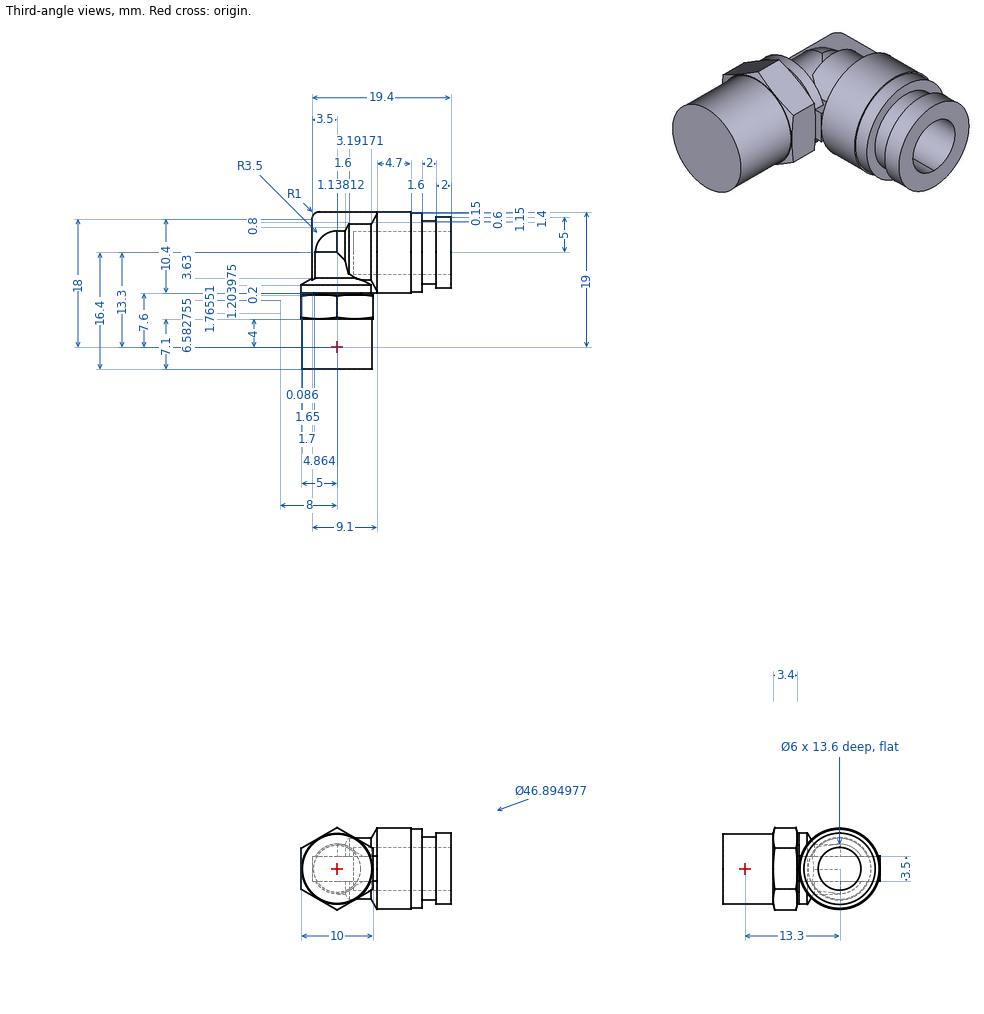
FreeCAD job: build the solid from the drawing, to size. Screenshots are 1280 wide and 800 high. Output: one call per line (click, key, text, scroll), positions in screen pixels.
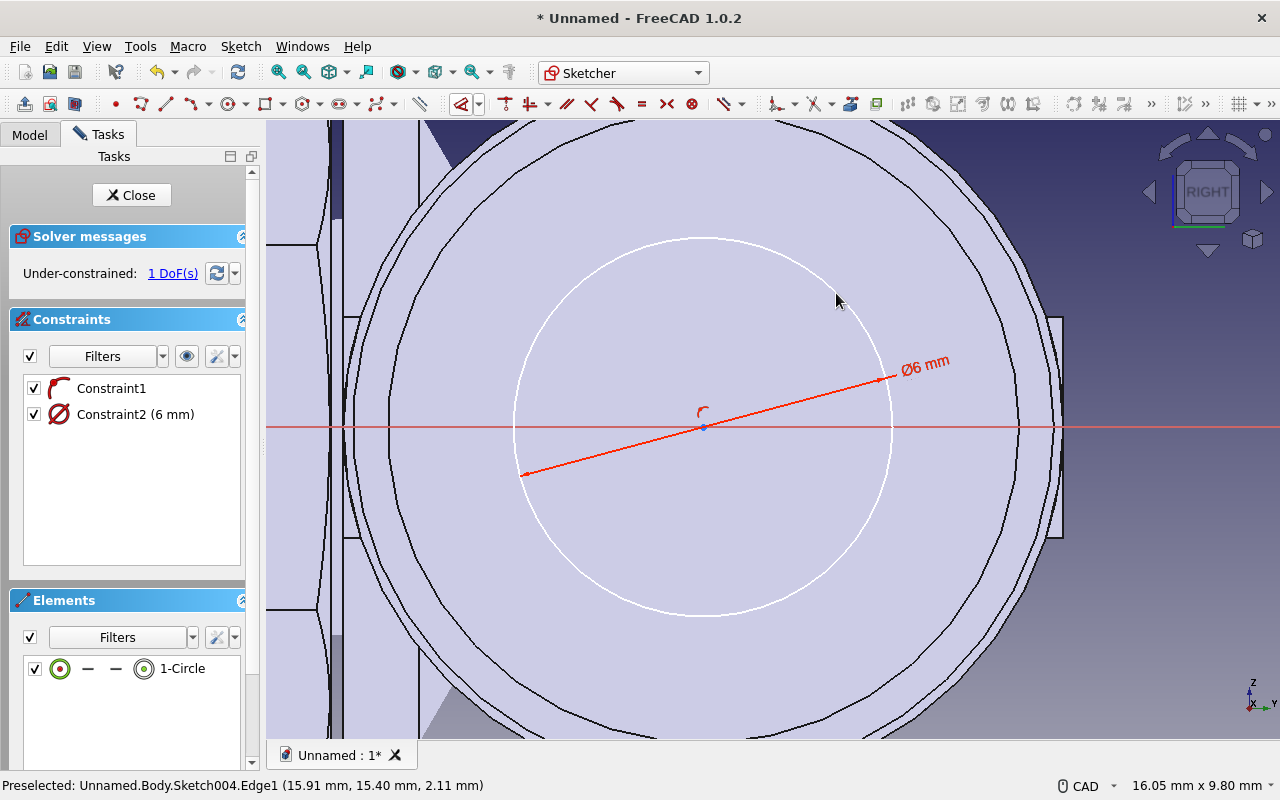
click(703, 427)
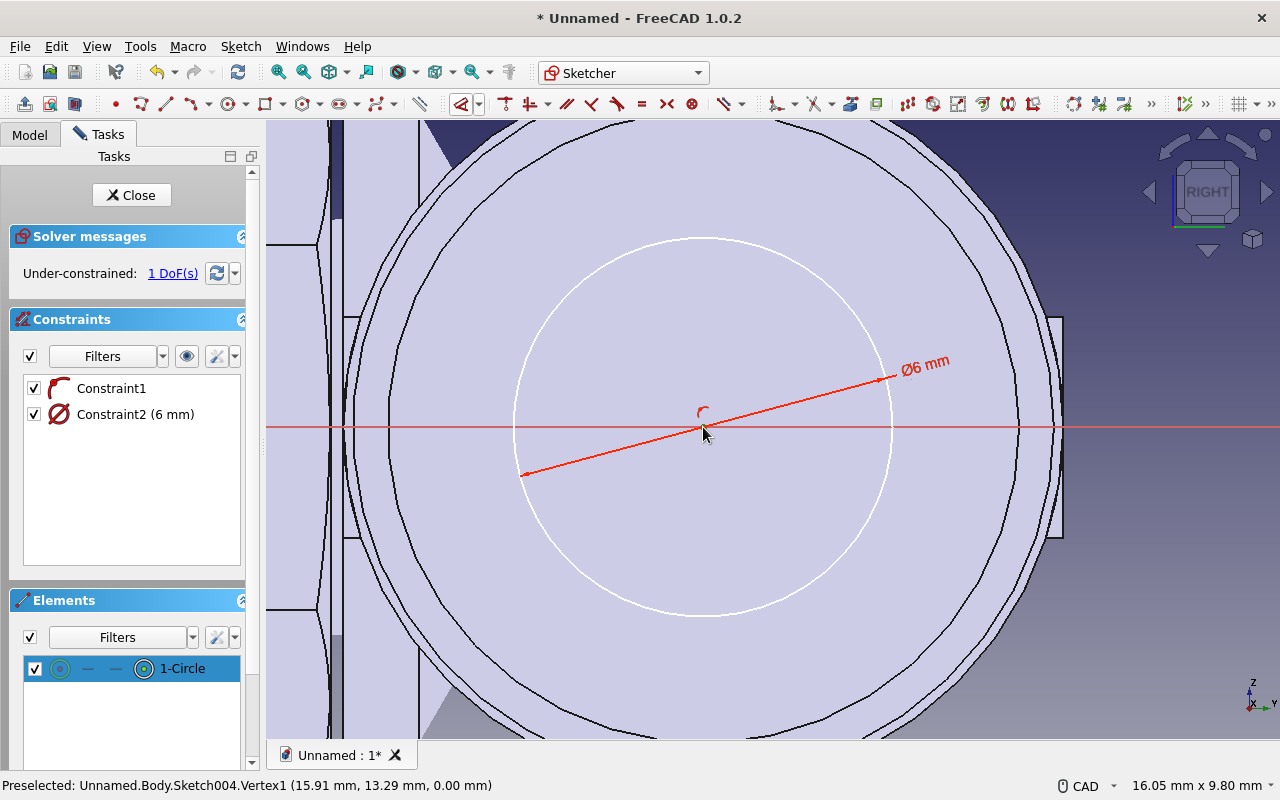
key(l)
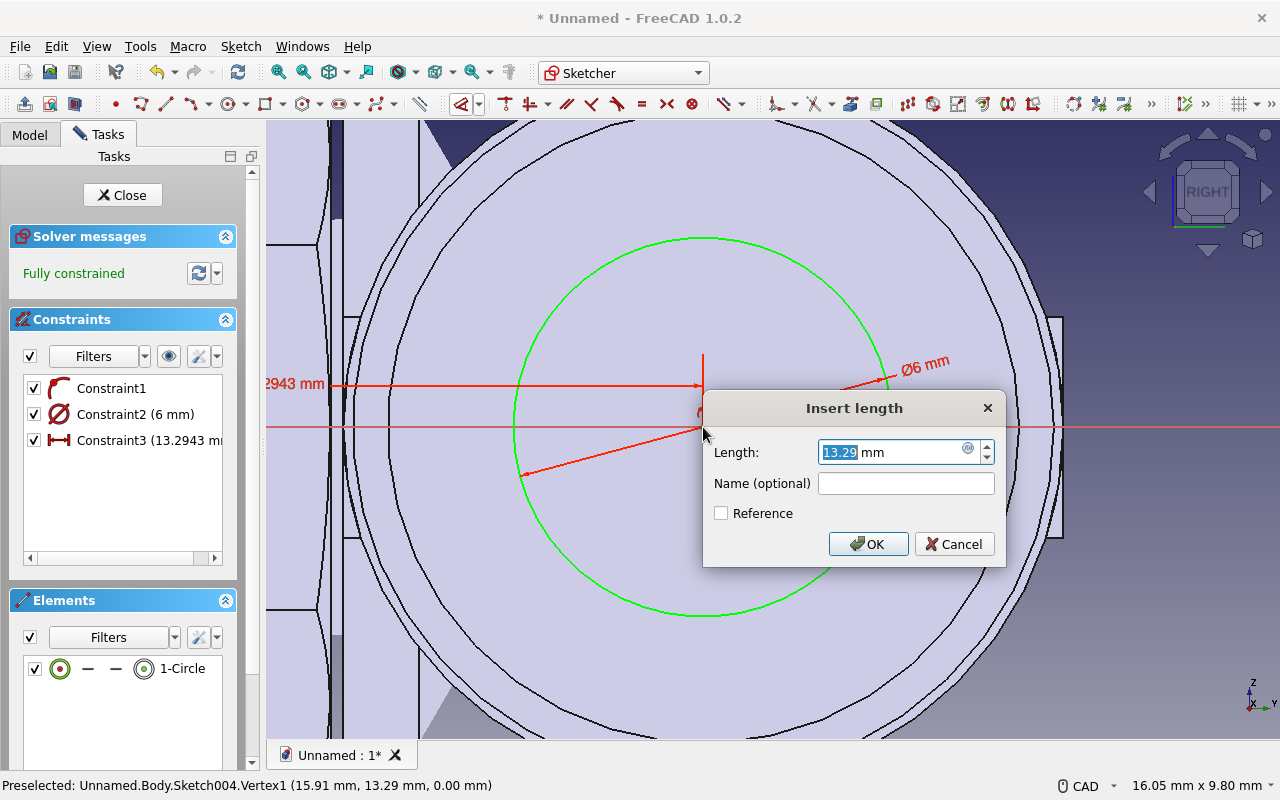
text(13.3)
key(Return)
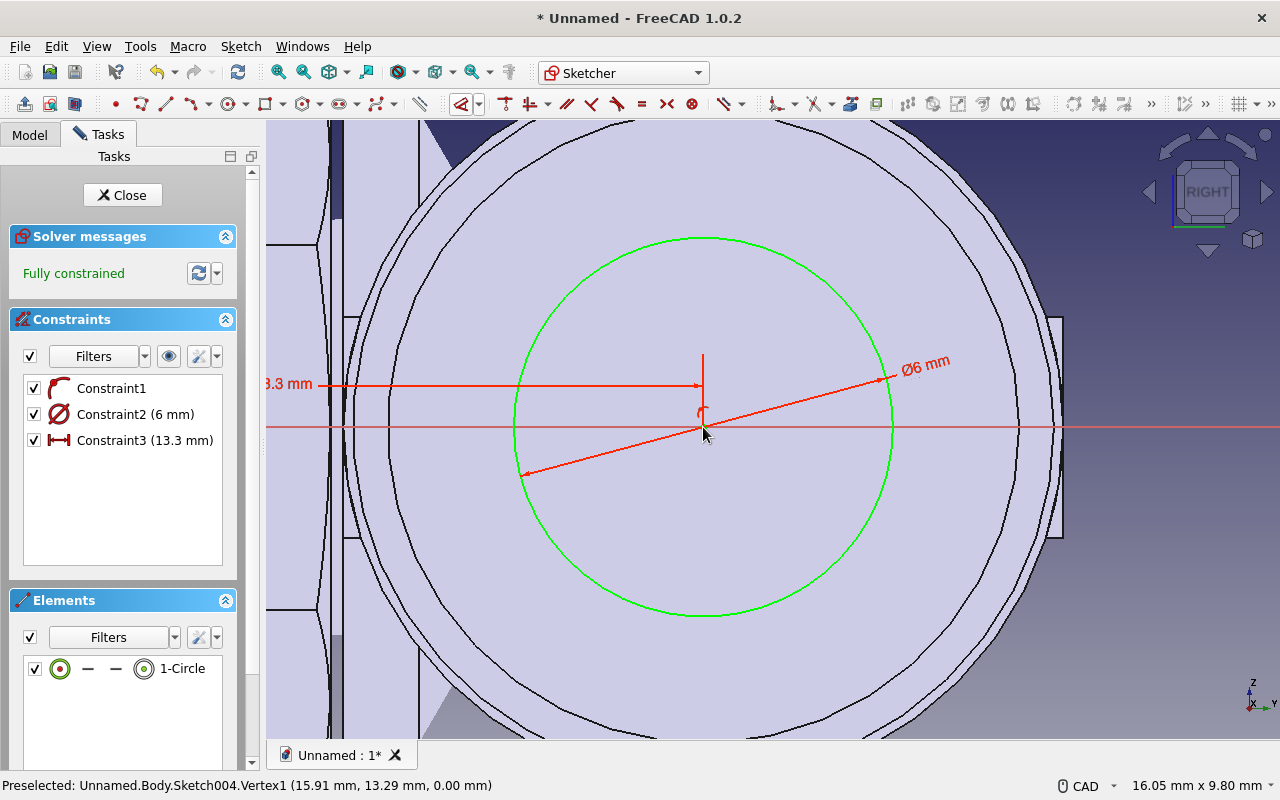
click(123, 195)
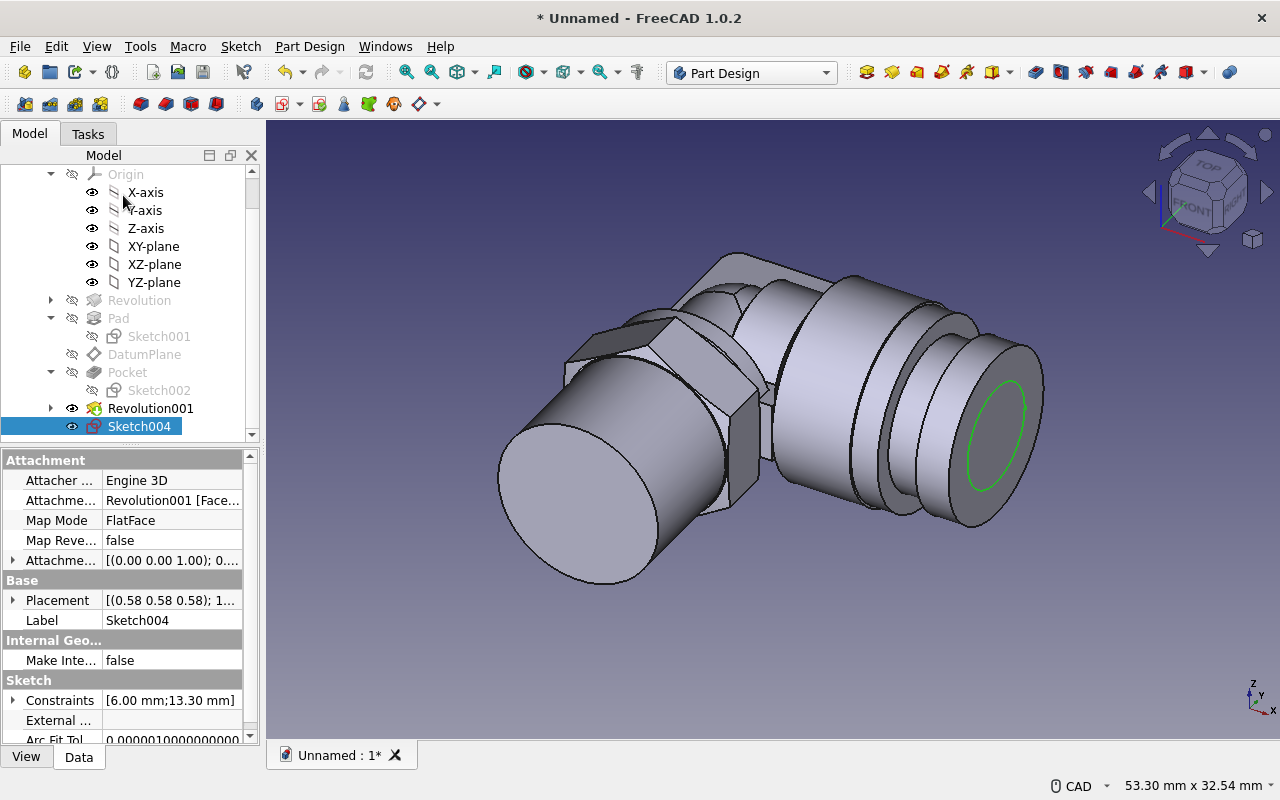
click(1061, 72)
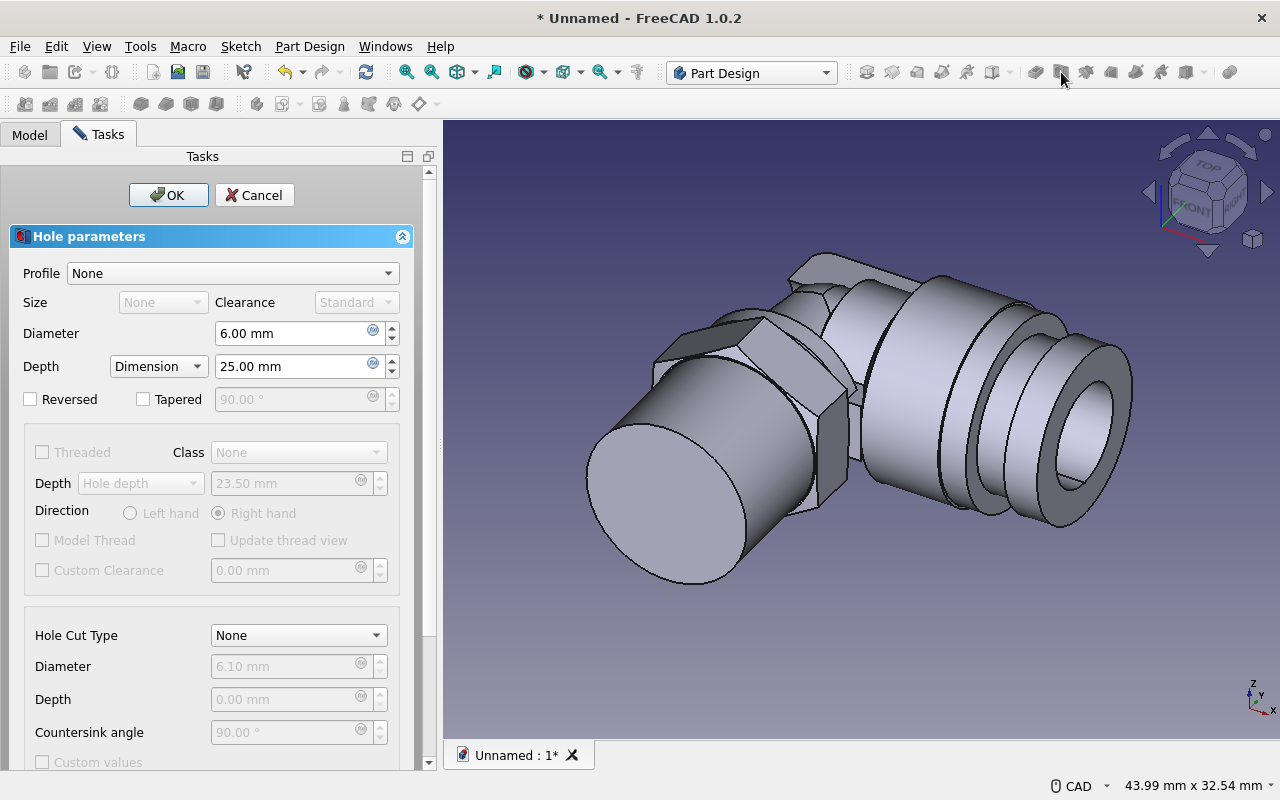
triple_click(300, 334)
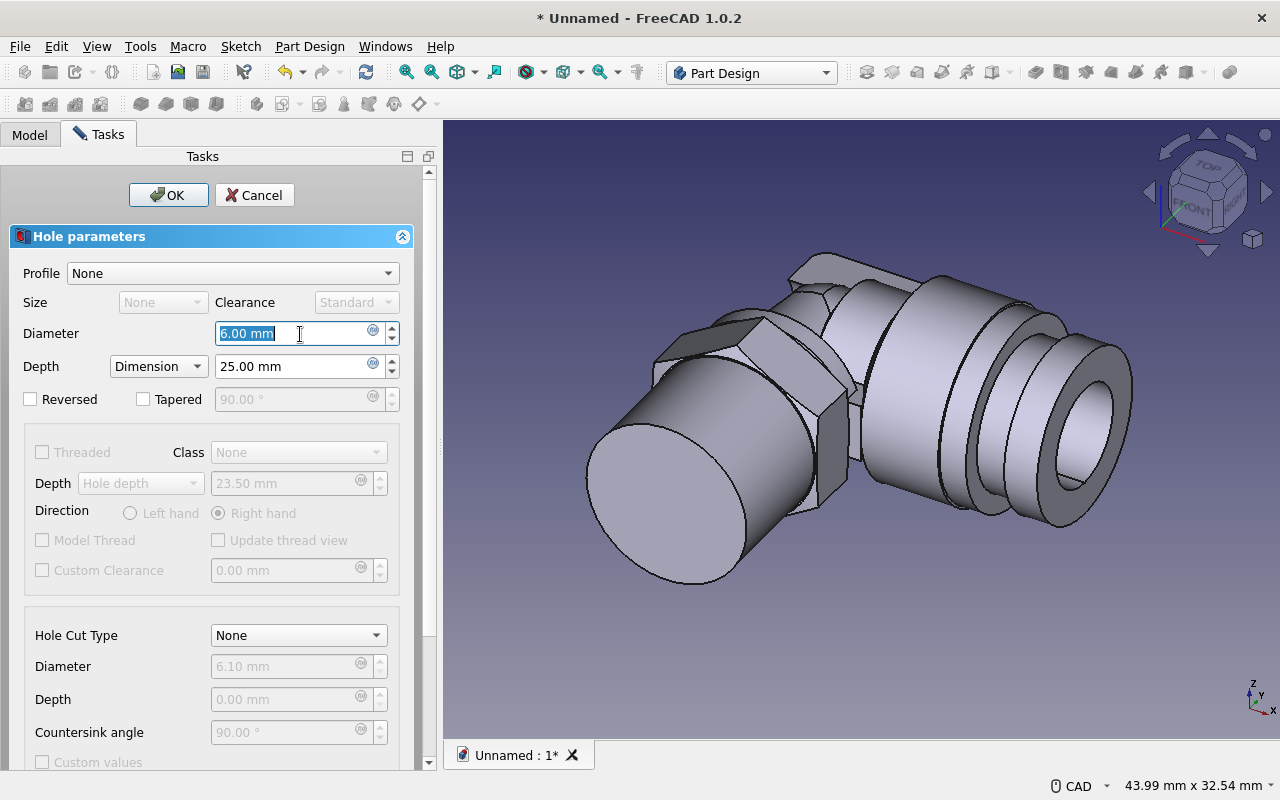
text(6)
key(Tab)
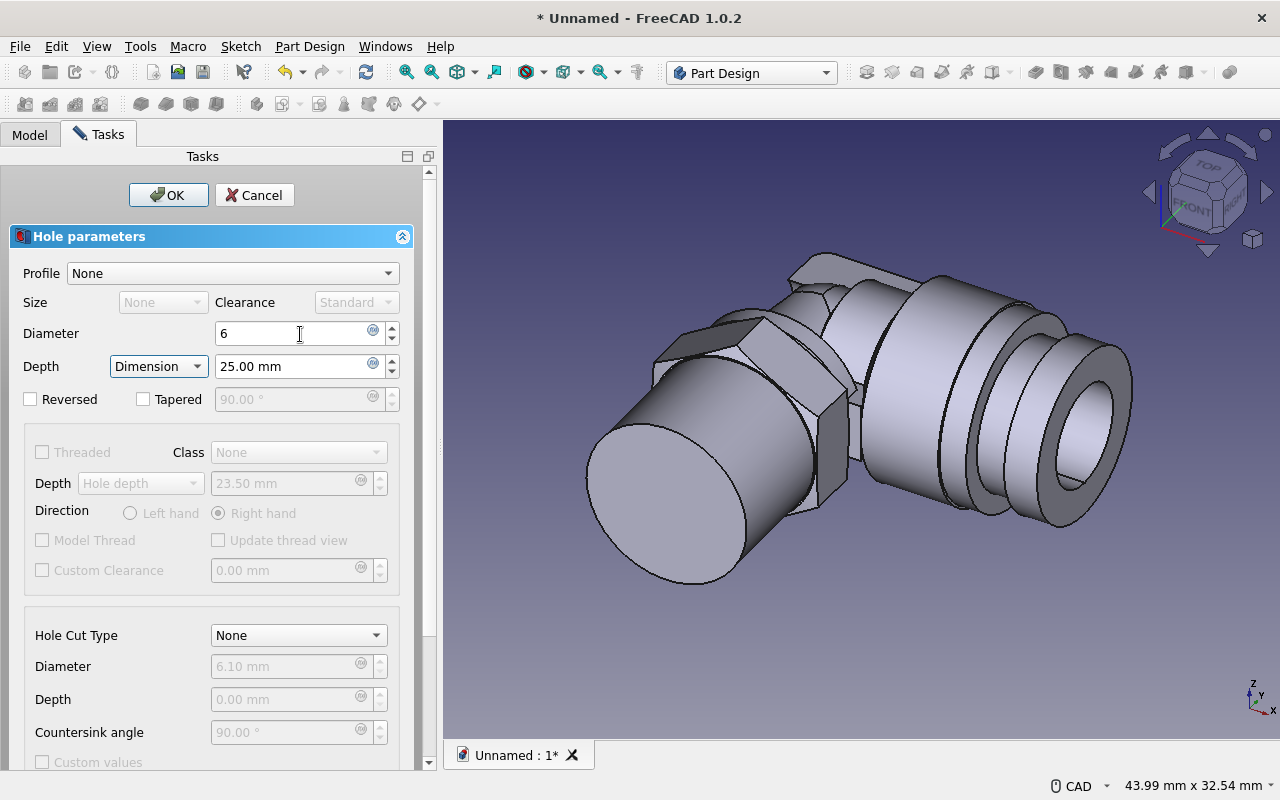
triple_click(300, 366)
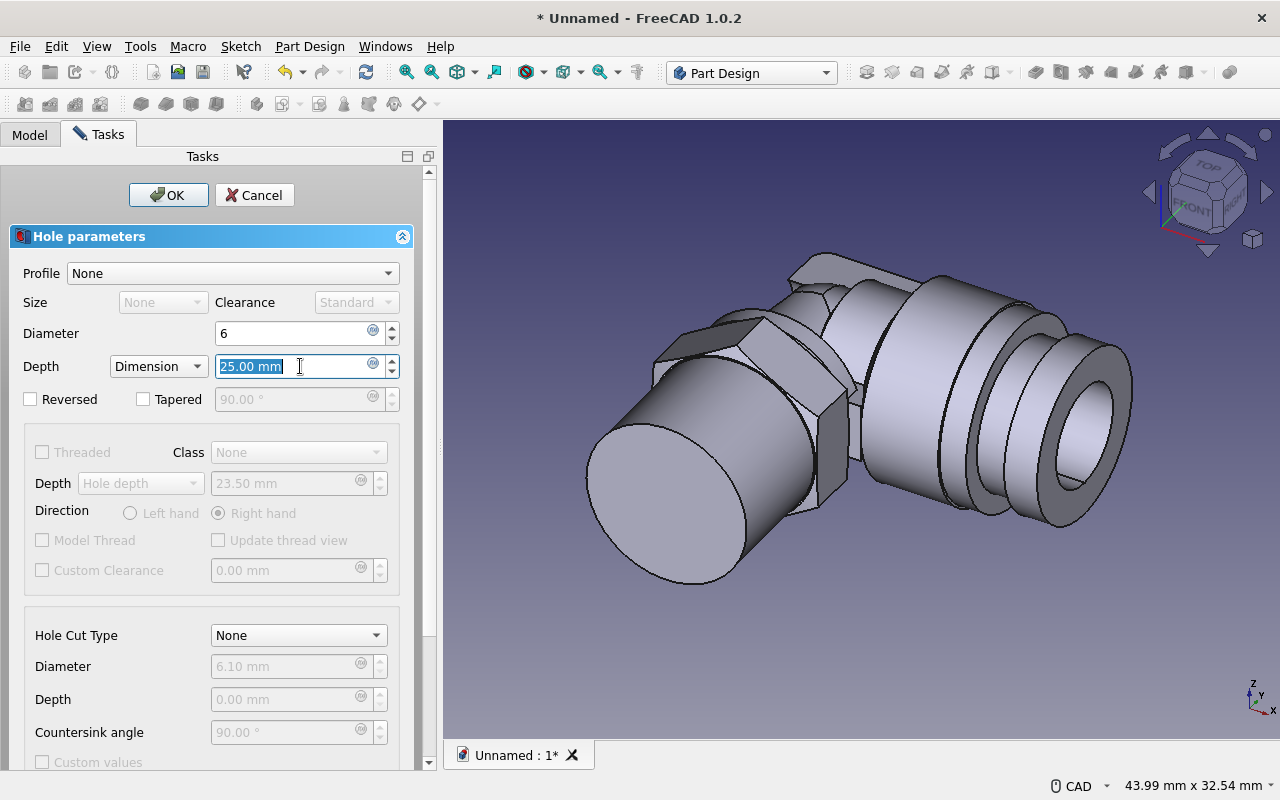
text(13.6)
key(Tab)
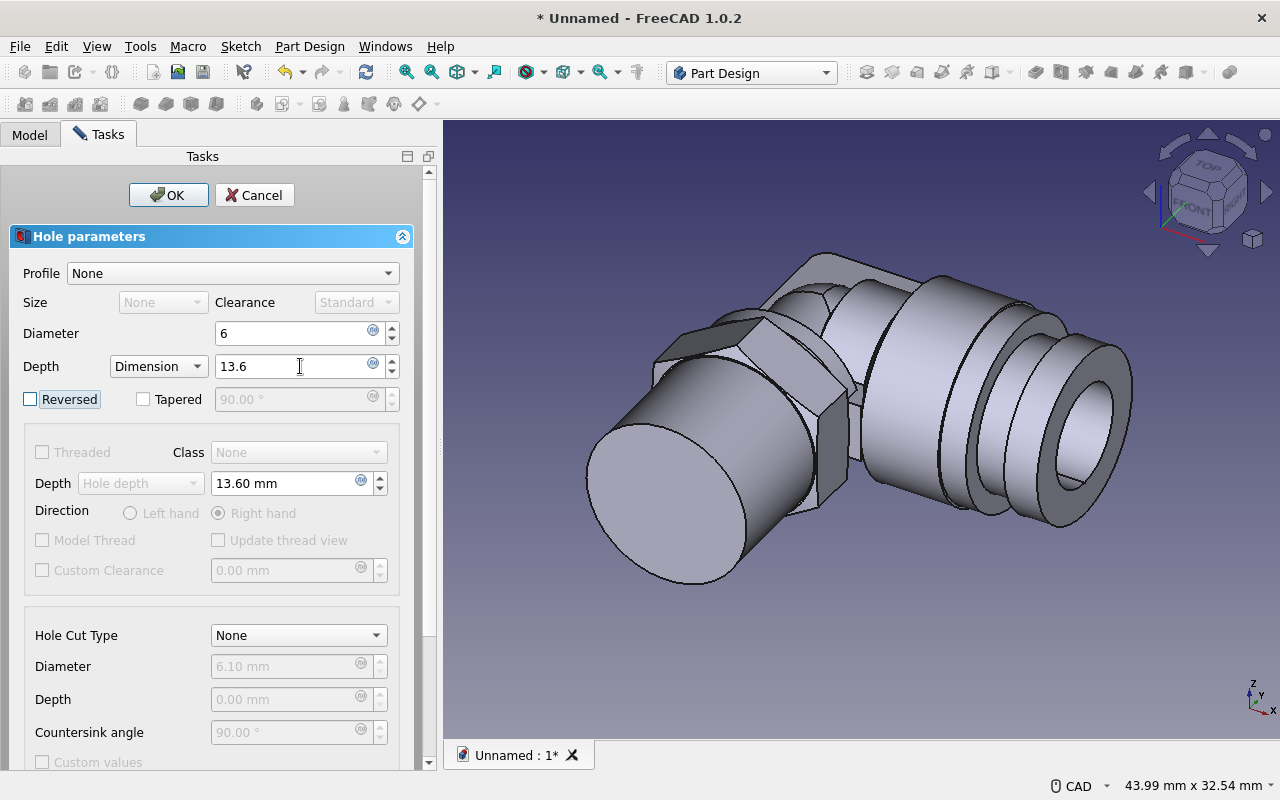
scroll(429, 468, down, 3)